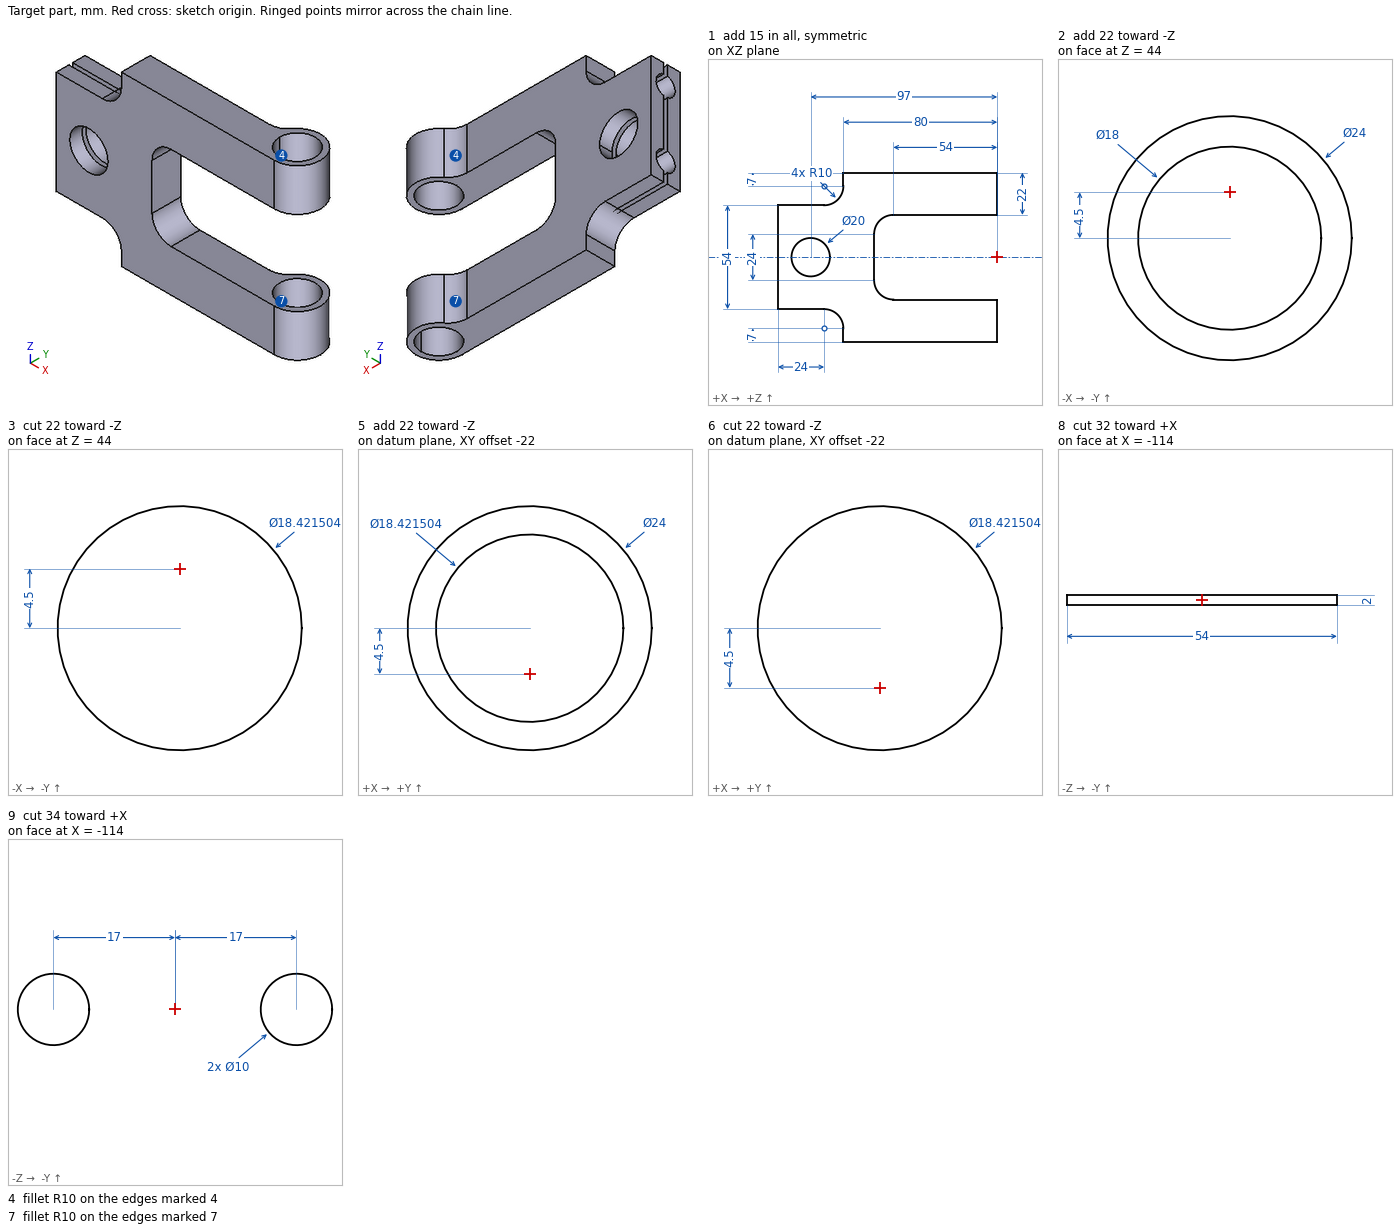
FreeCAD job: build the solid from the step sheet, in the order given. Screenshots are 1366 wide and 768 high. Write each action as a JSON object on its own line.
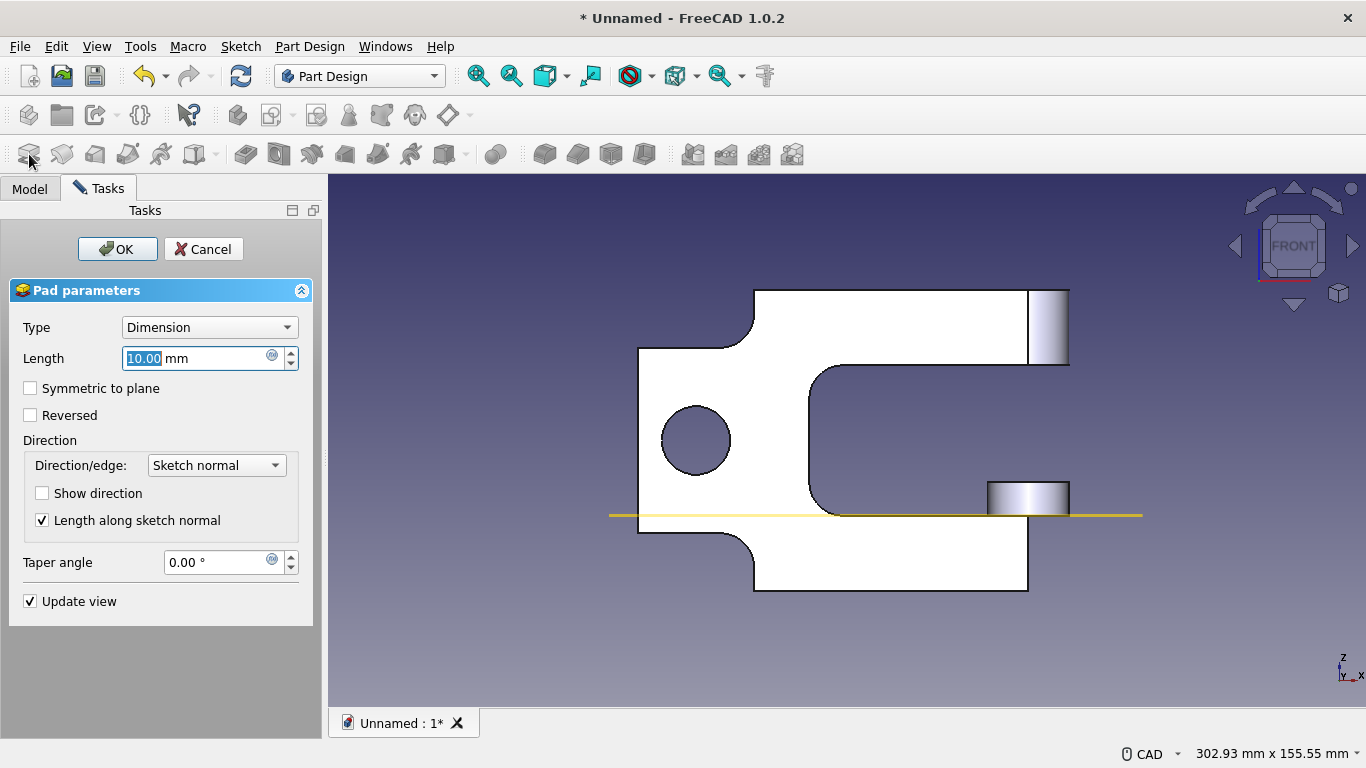
{"action": "type", "text": "22"}
{"action": "key", "text": "Tab"}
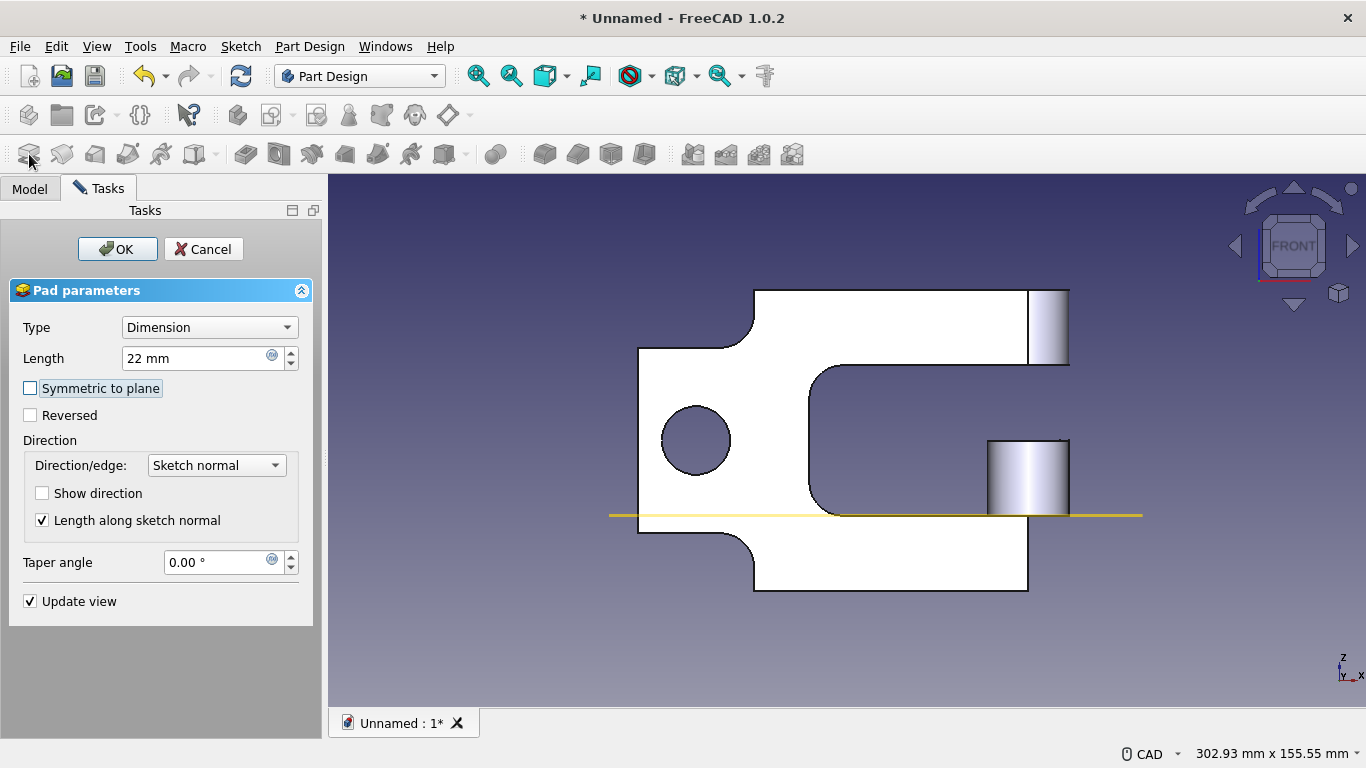
{"action": "left_click", "coordinate": [31, 415]}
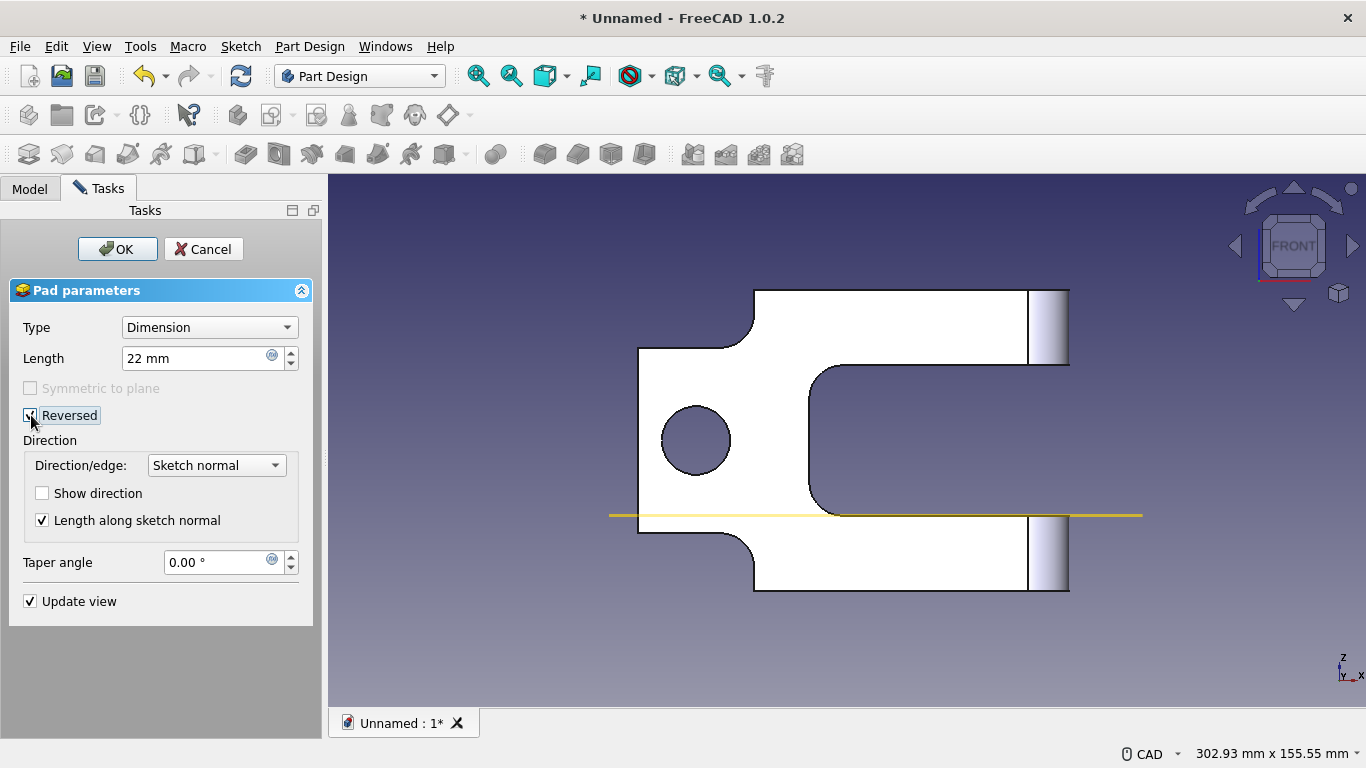
{"action": "left_click", "coordinate": [118, 249]}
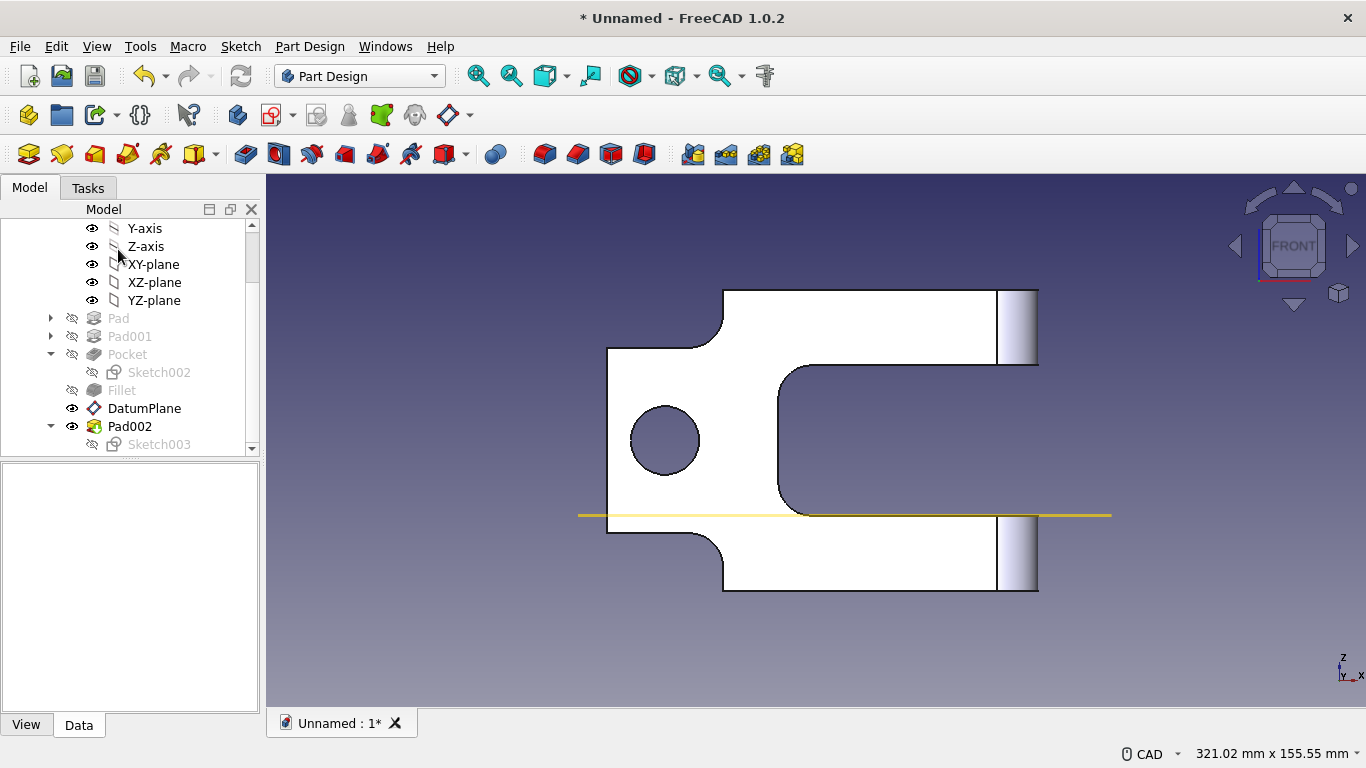
{"action": "left_click", "coordinate": [117, 408]}
{"action": "key", "text": "space"}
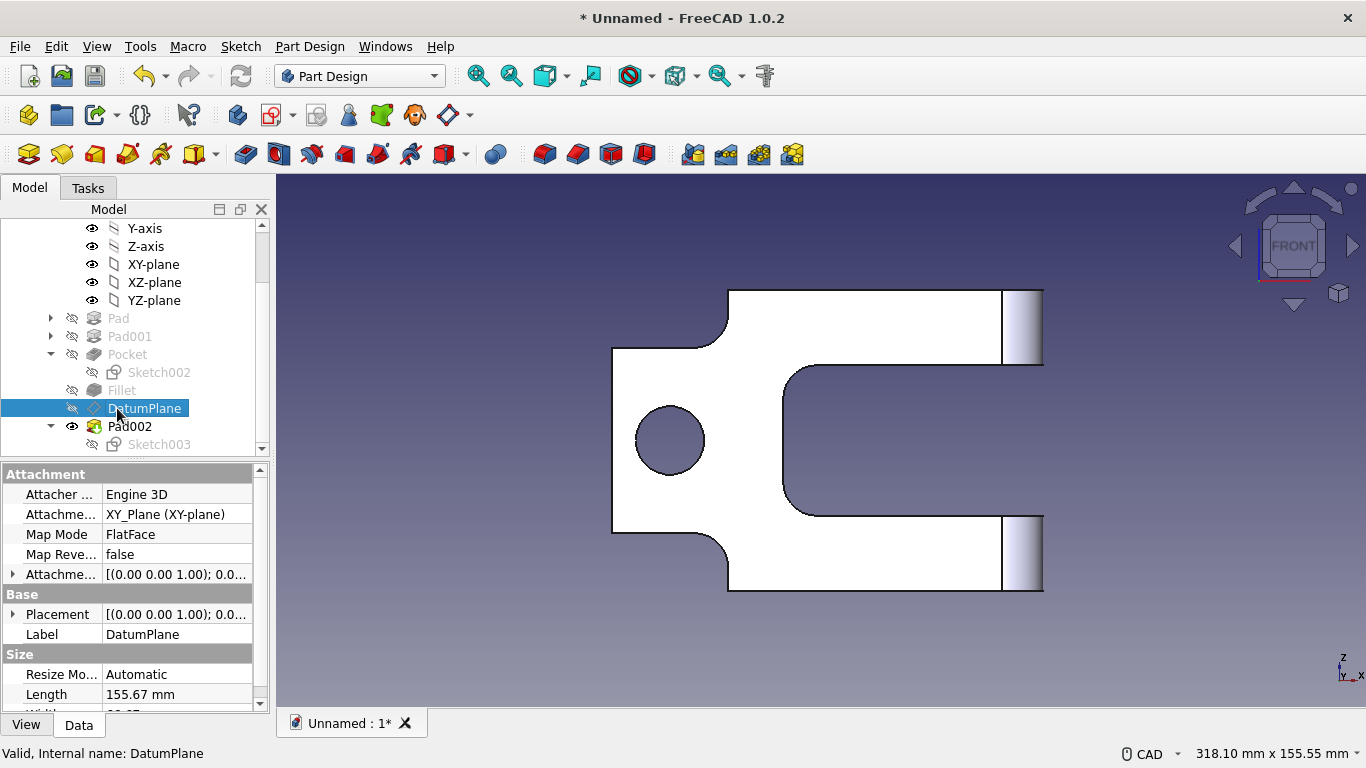
{"action": "scroll", "coordinate": [161, 332], "scroll_direction": "down", "scroll_amount": 3}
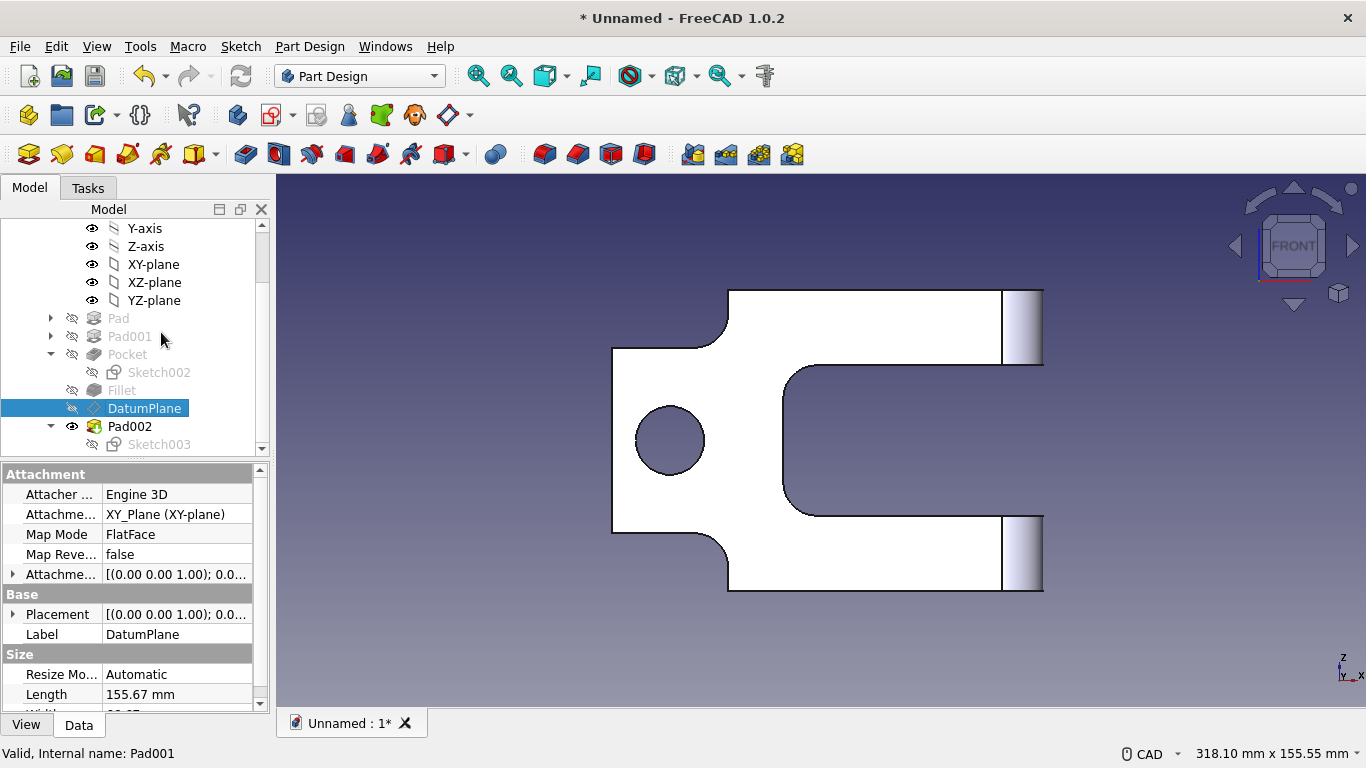
{"action": "scroll", "coordinate": [161, 332], "scroll_direction": "up", "scroll_amount": 15}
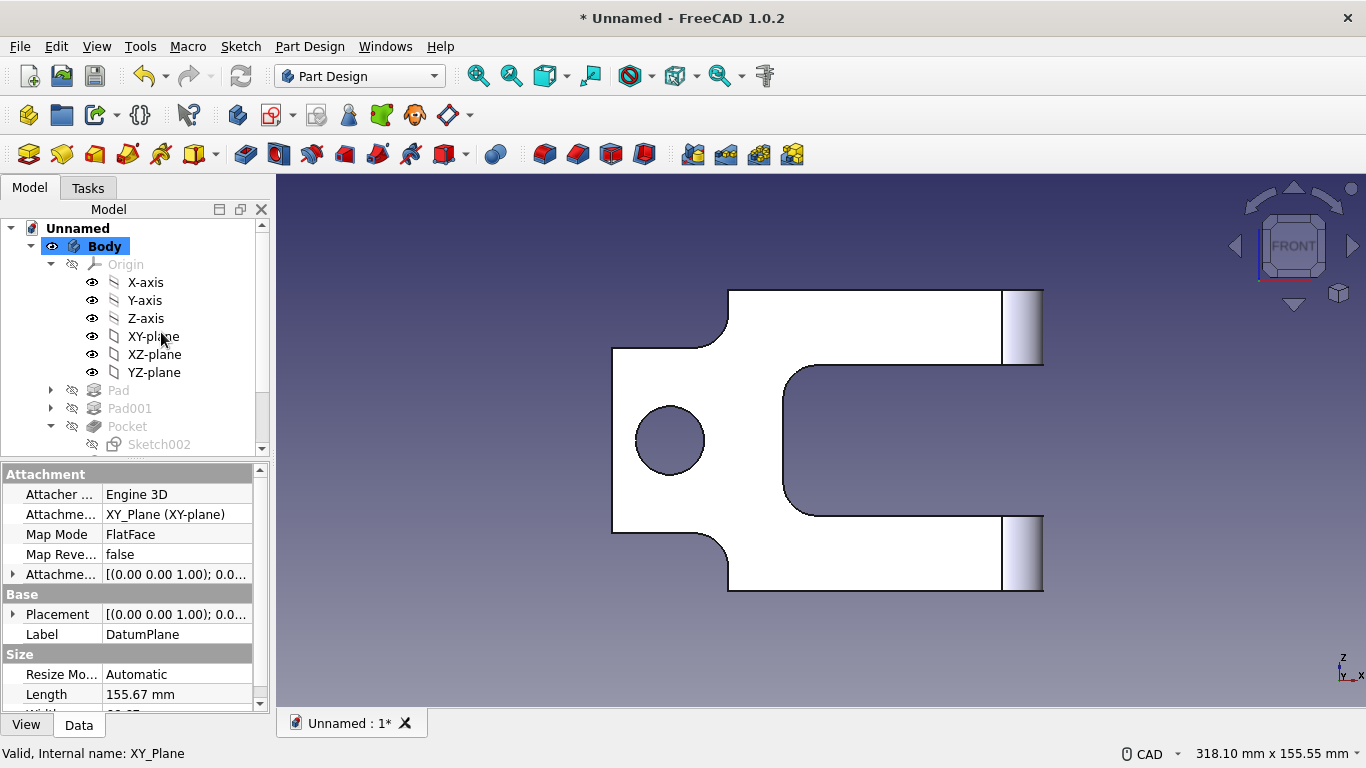
{"action": "left_click", "coordinate": [137, 336]}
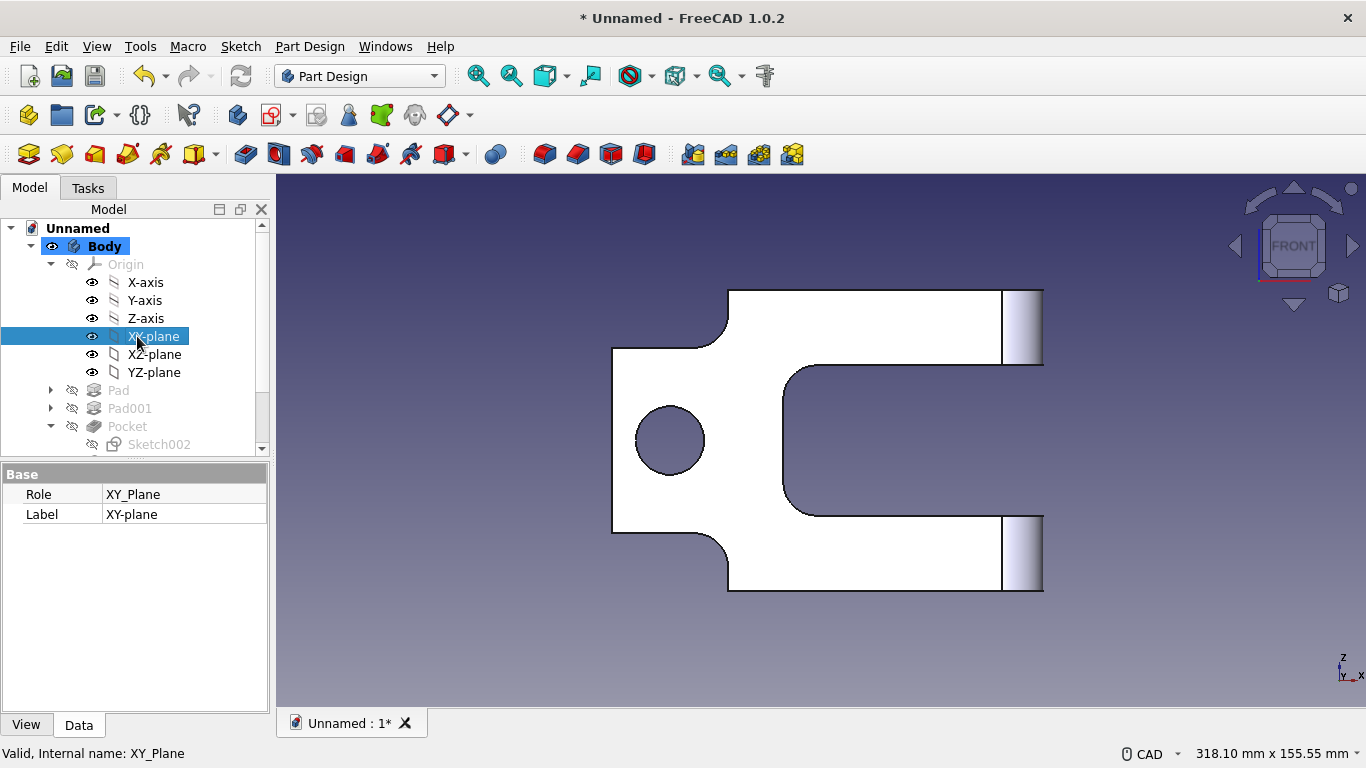
{"action": "left_click", "coordinate": [448, 116]}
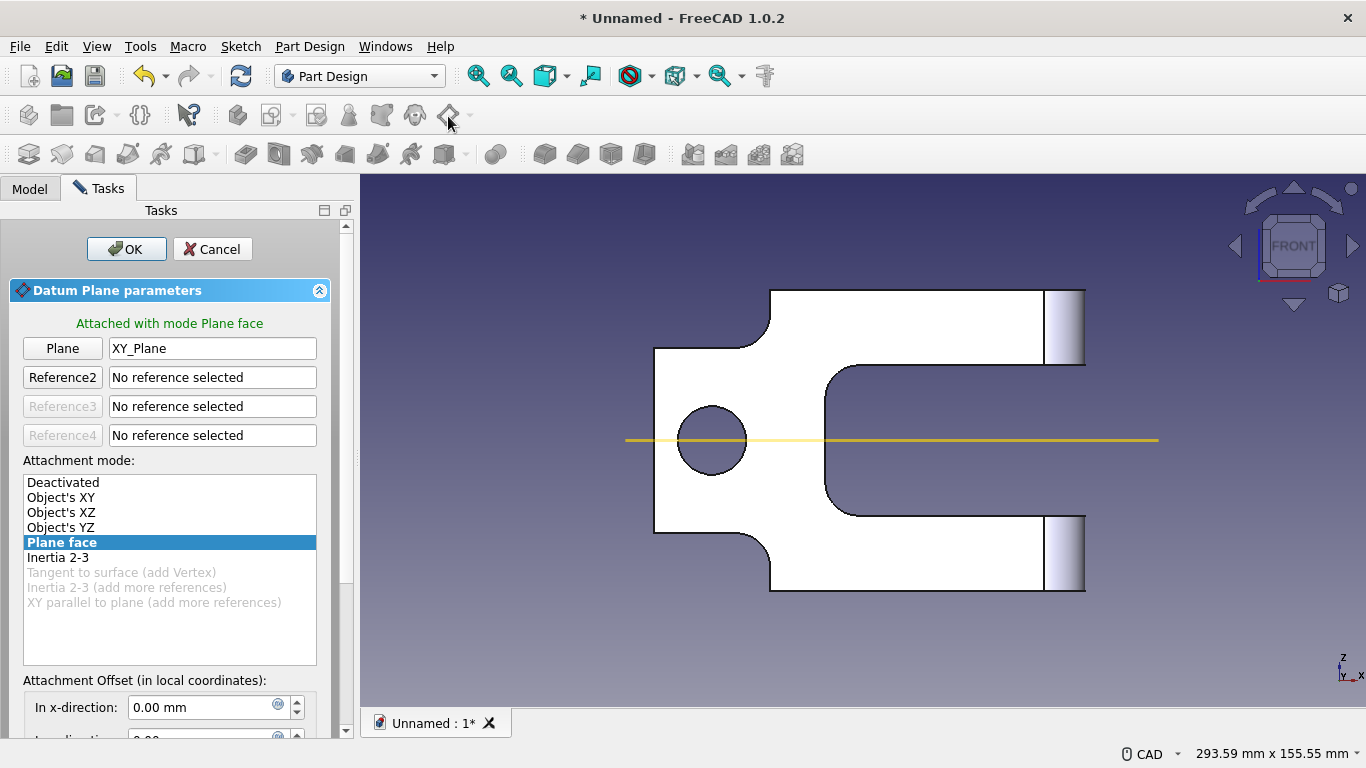
{"action": "scroll", "coordinate": [346, 479], "scroll_direction": "down", "scroll_amount": 2}